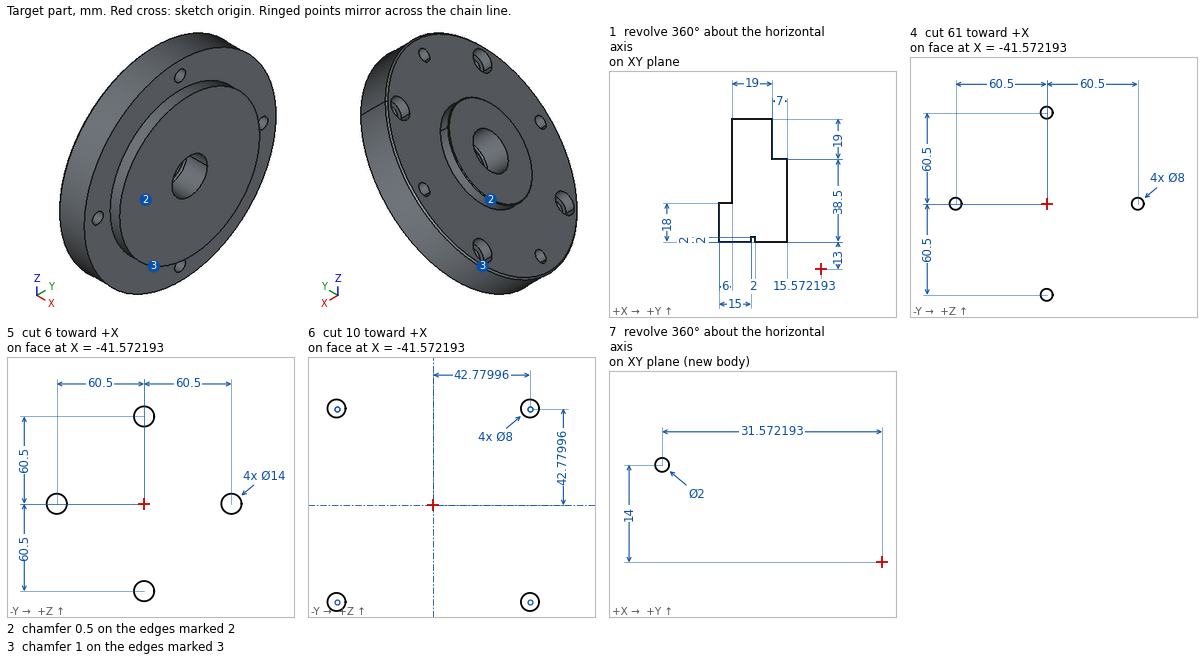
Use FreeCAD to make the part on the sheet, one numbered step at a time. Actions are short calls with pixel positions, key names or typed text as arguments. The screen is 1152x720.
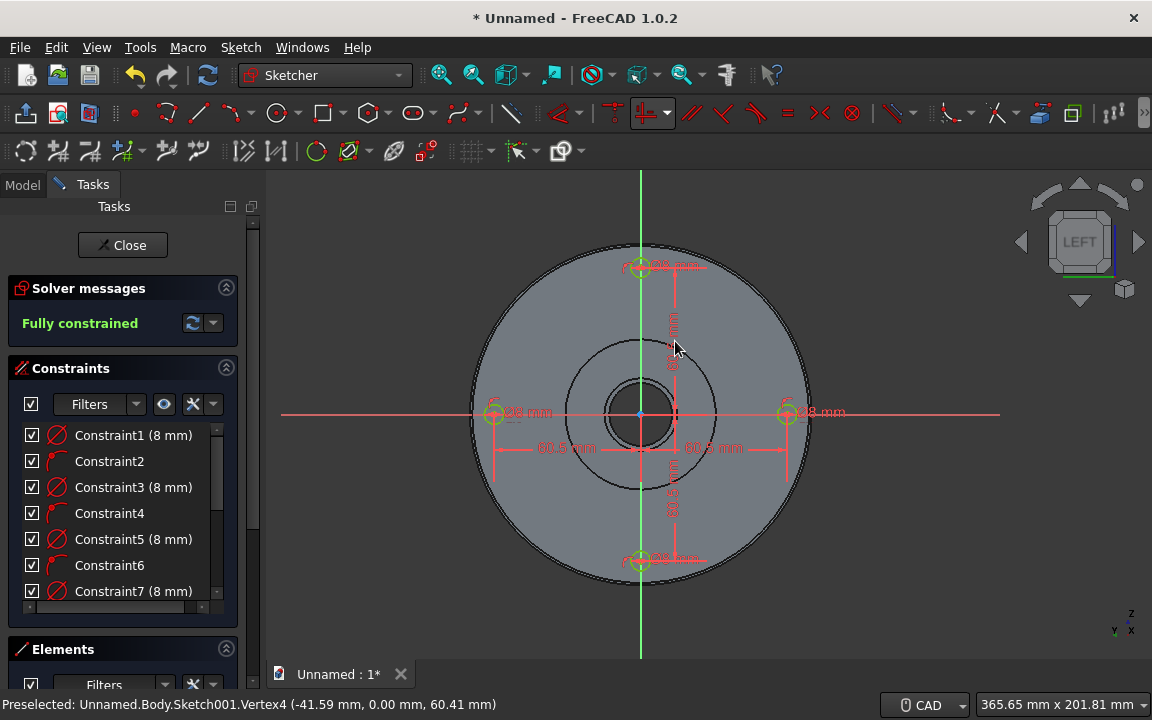
click(123, 245)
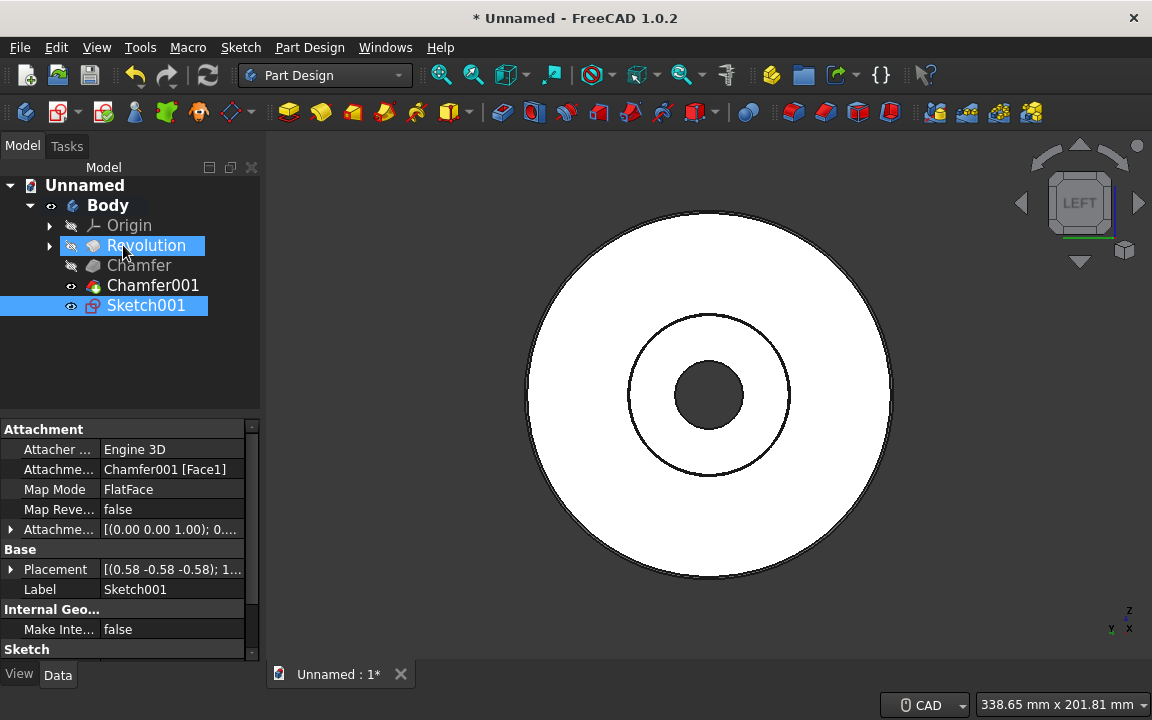
click(504, 112)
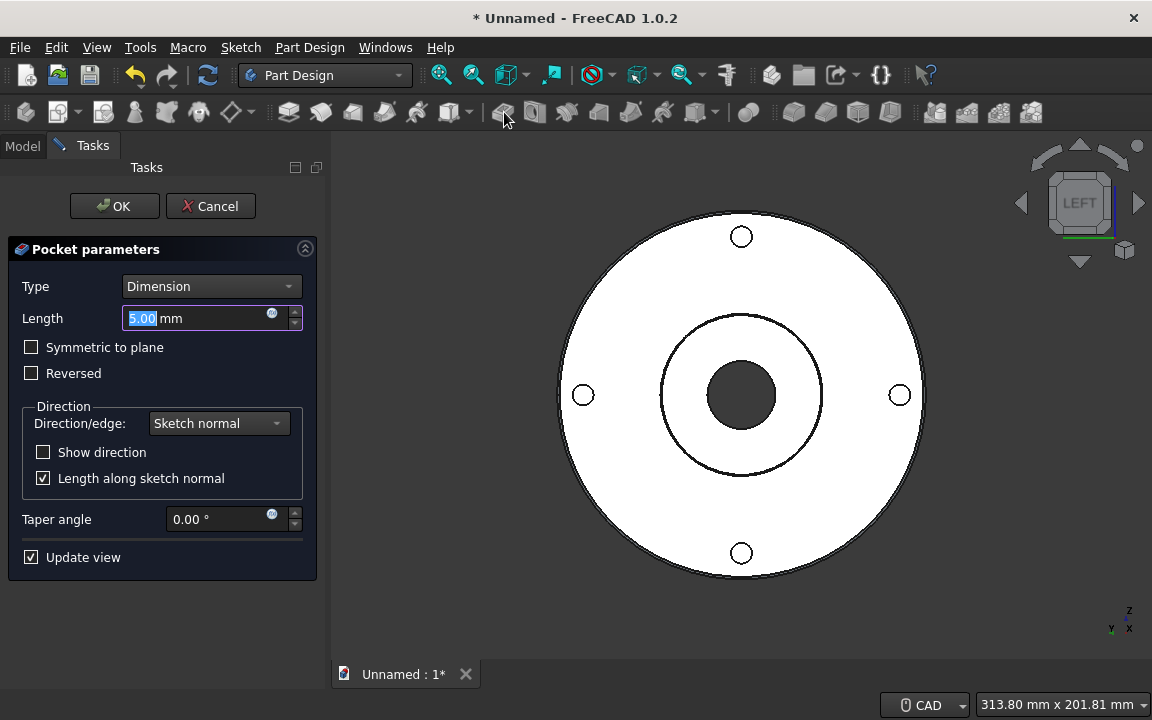
text(61)
key(Tab)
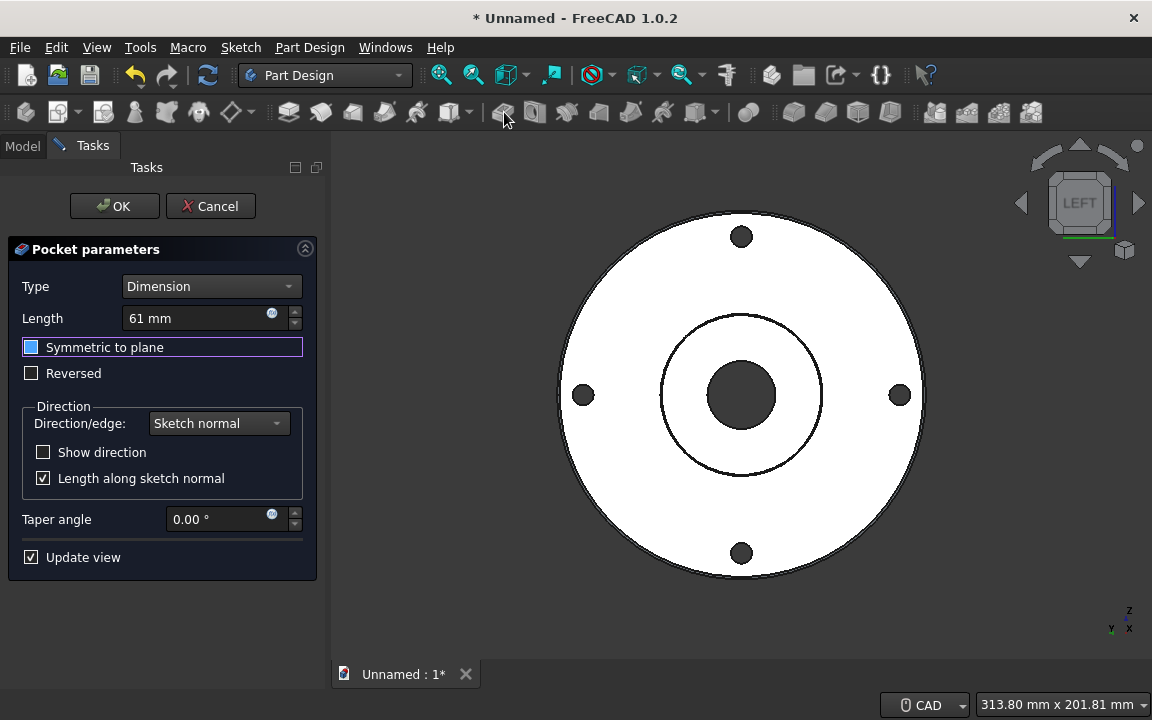
click(115, 206)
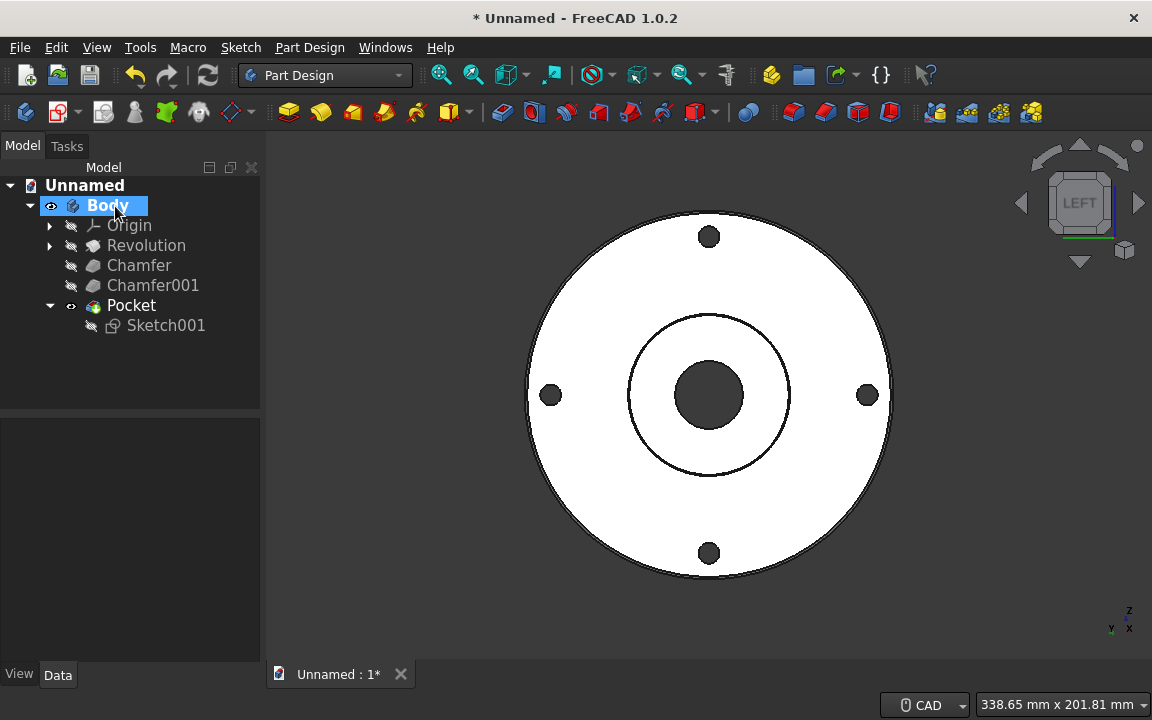
click(657, 498)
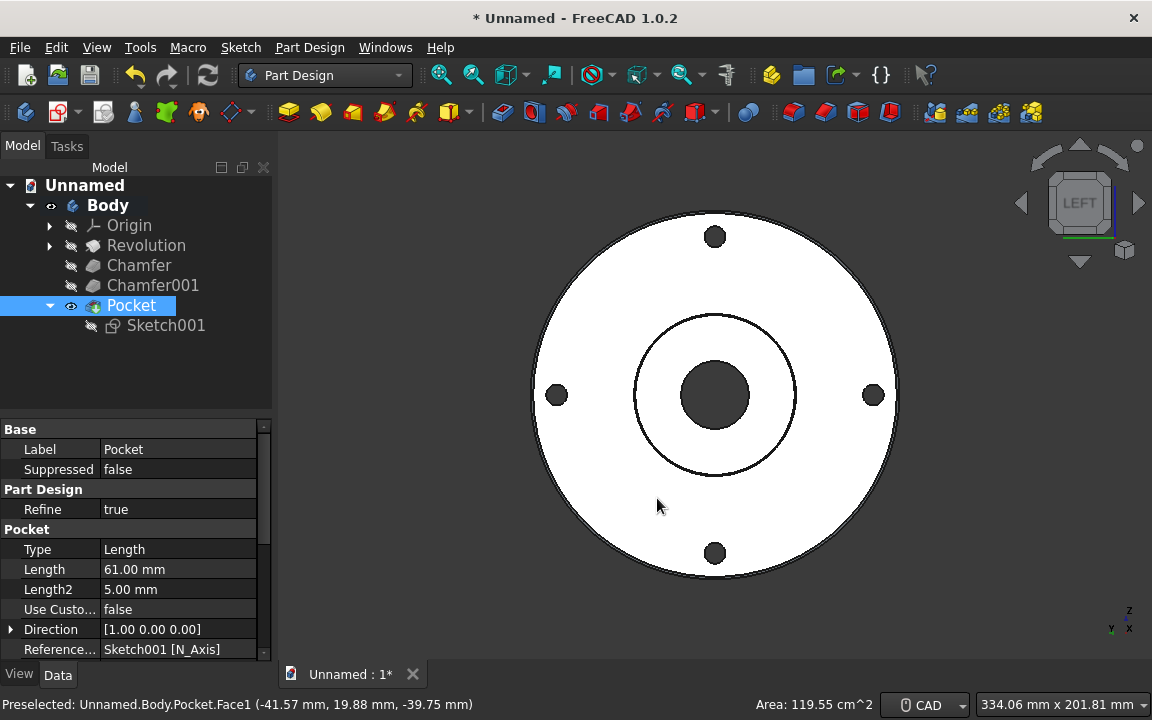
click(58, 112)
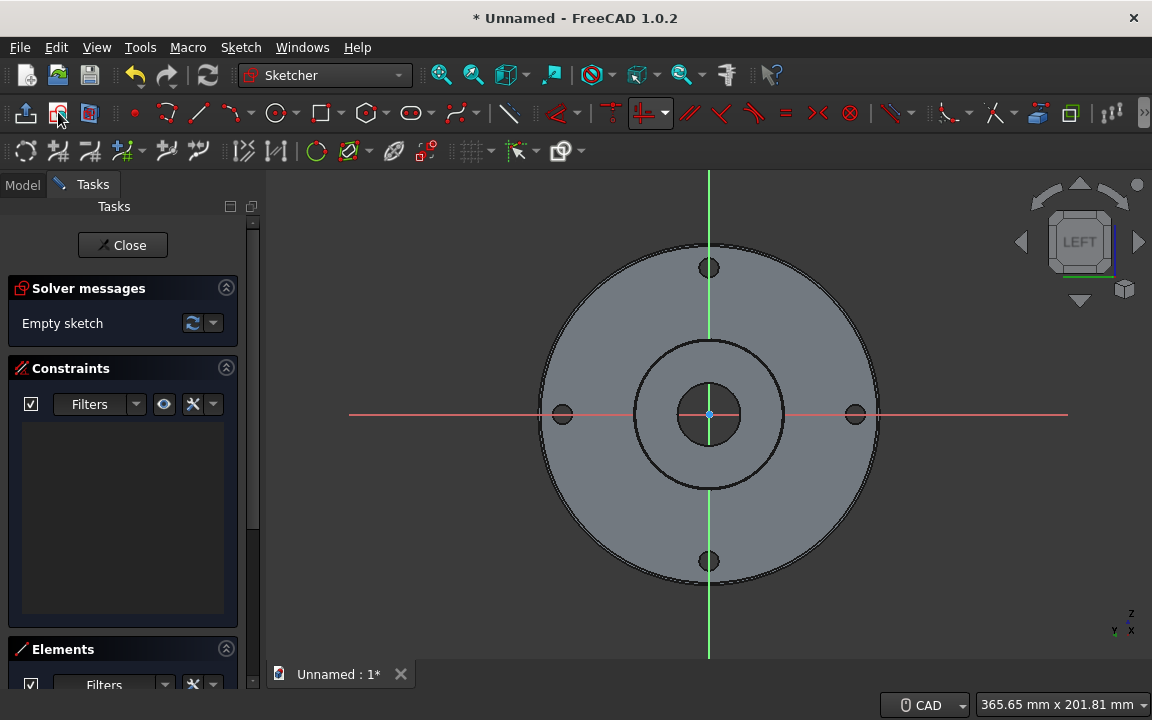
click(276, 114)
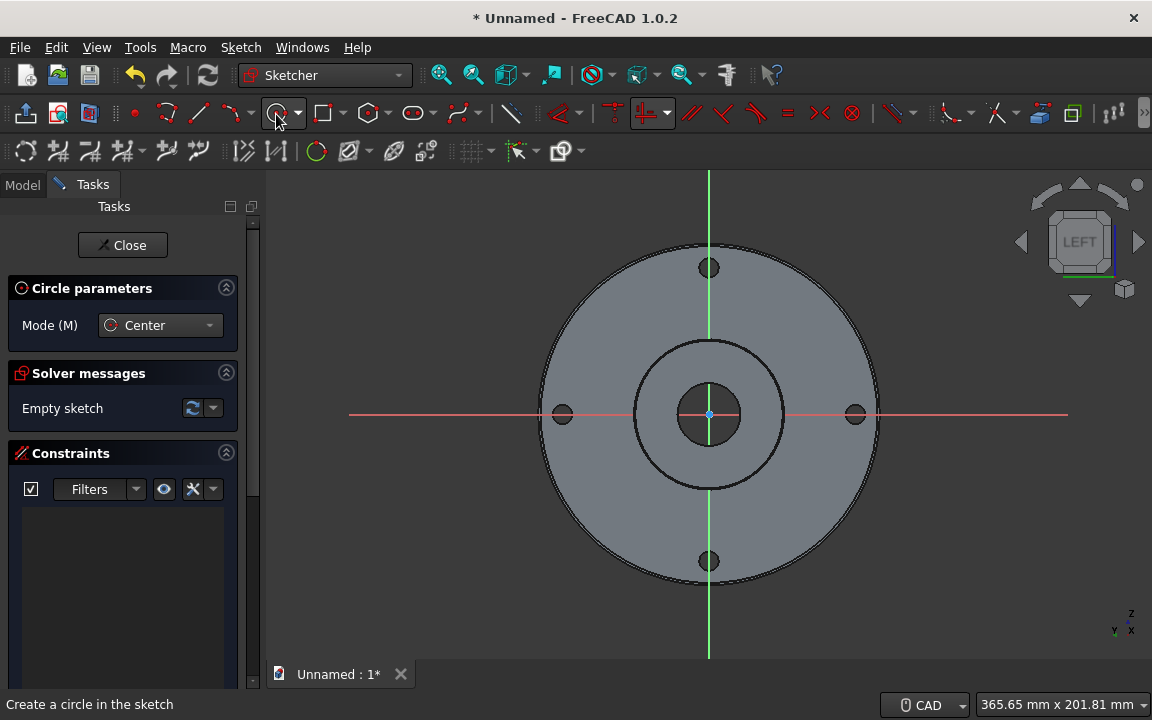
scroll(856, 415, up, 2)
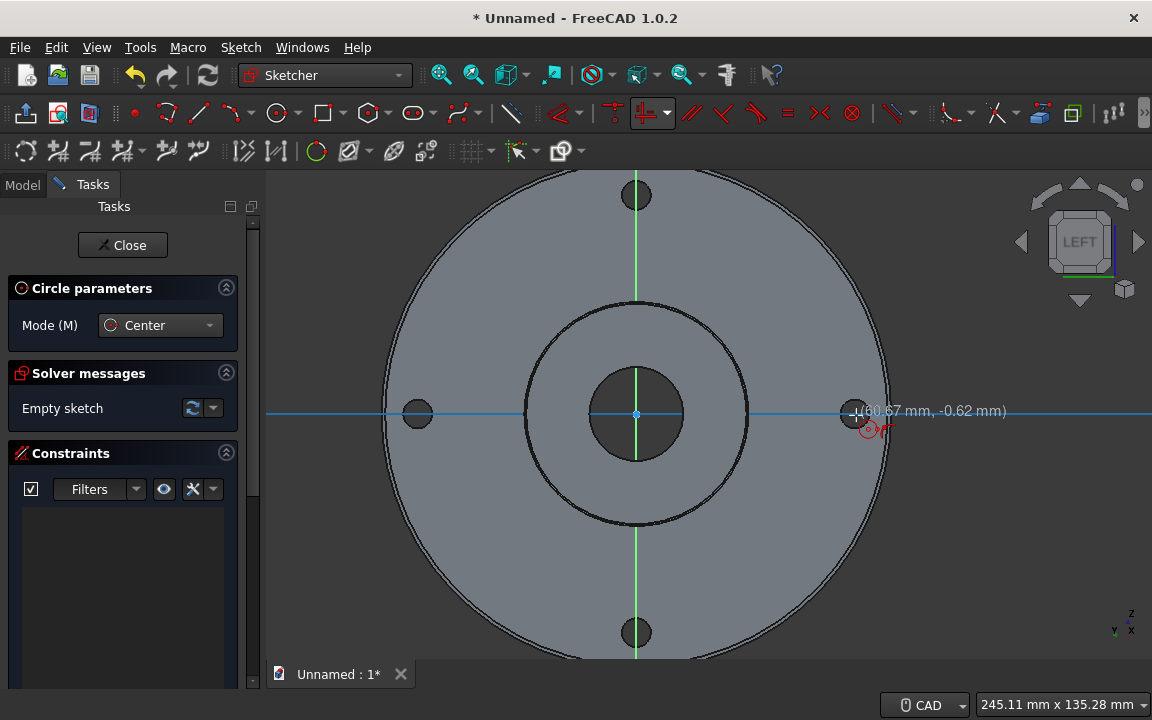
click(855, 414)
move(873, 396)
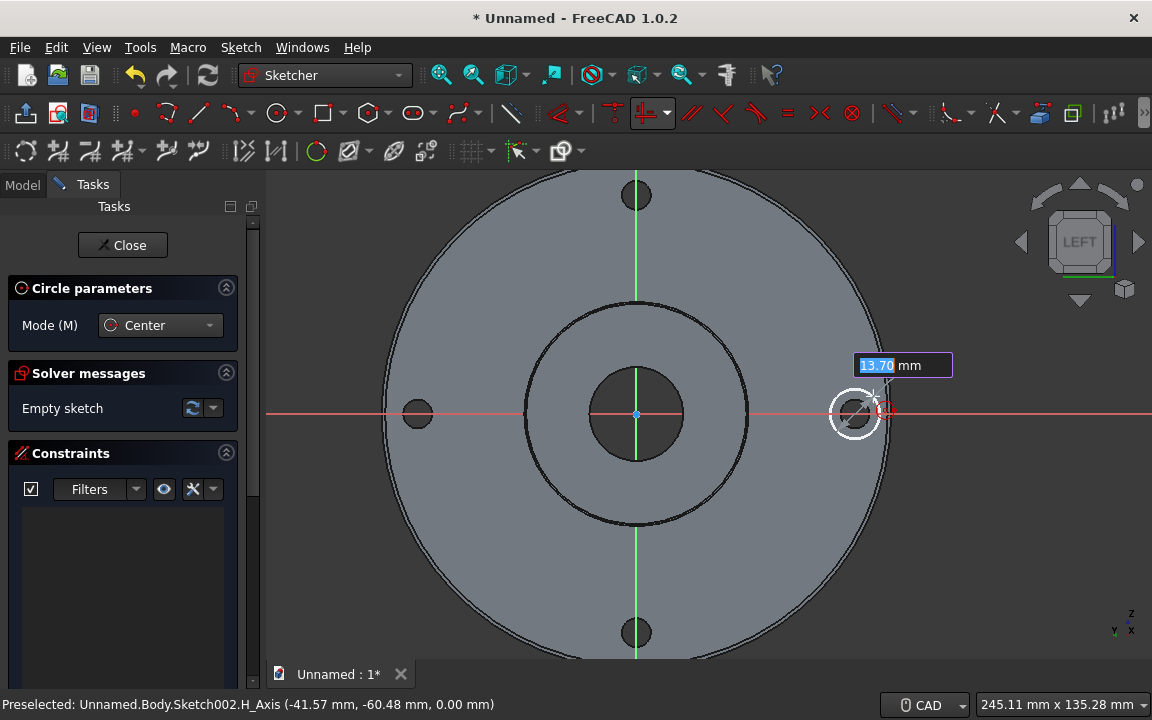
text(14)
key(Return)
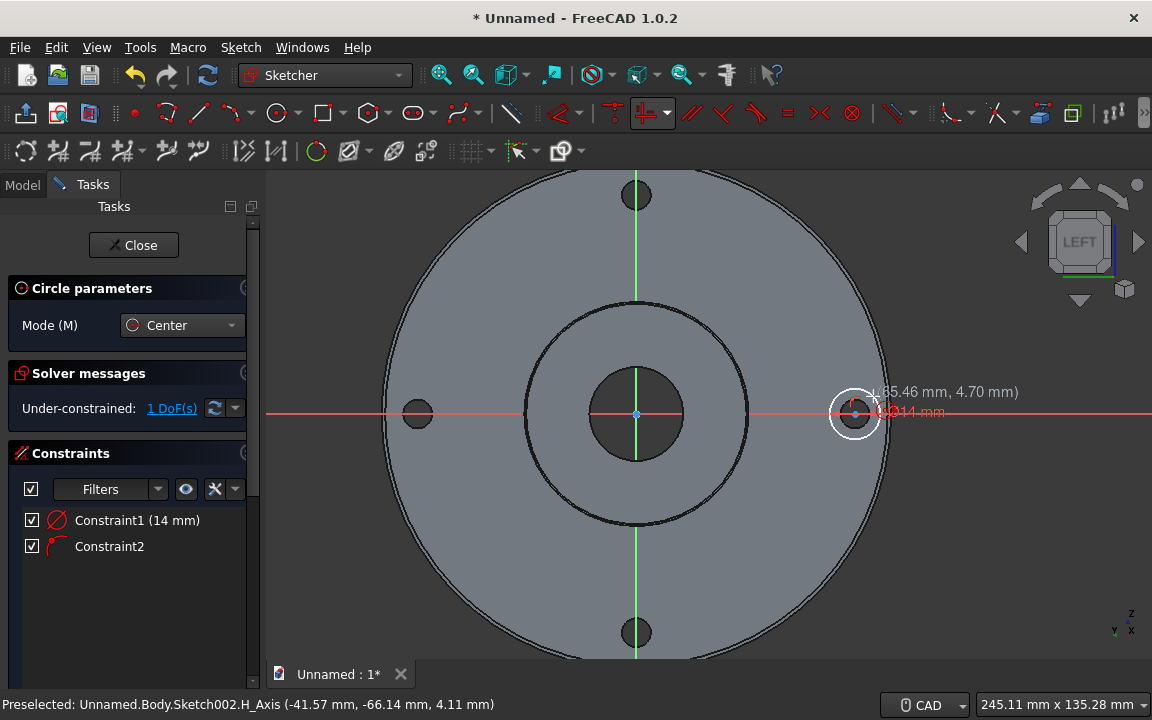
scroll(649, 416, down, 2)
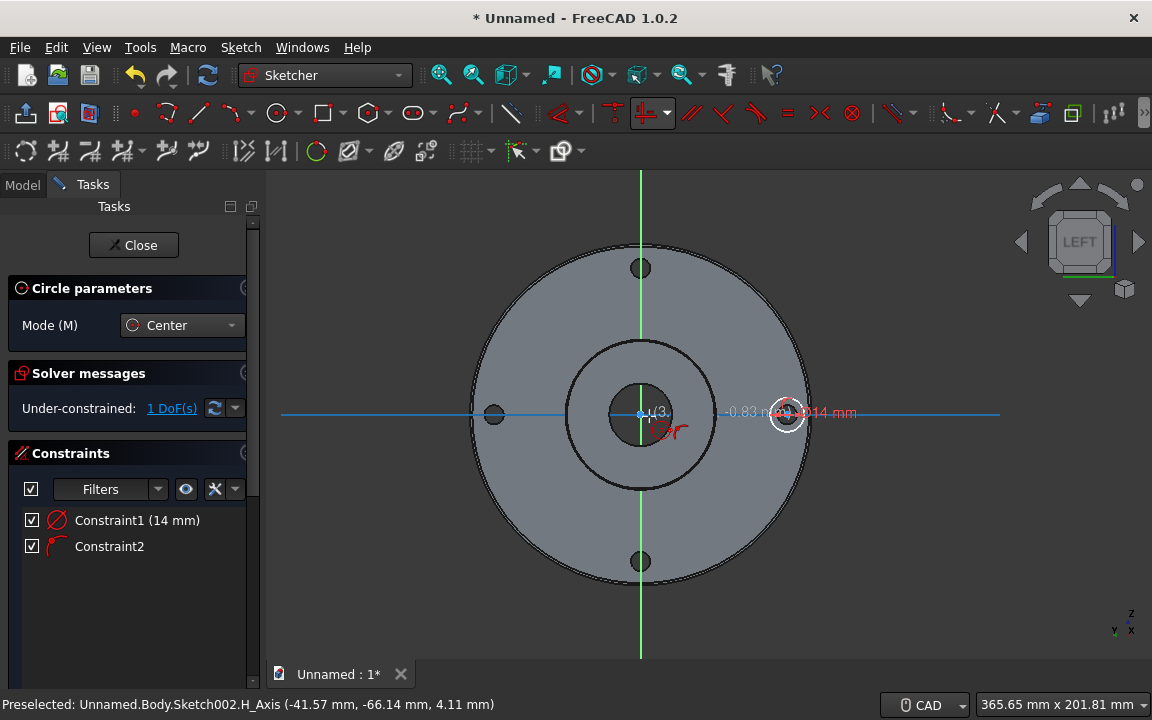
scroll(641, 561, up, 2)